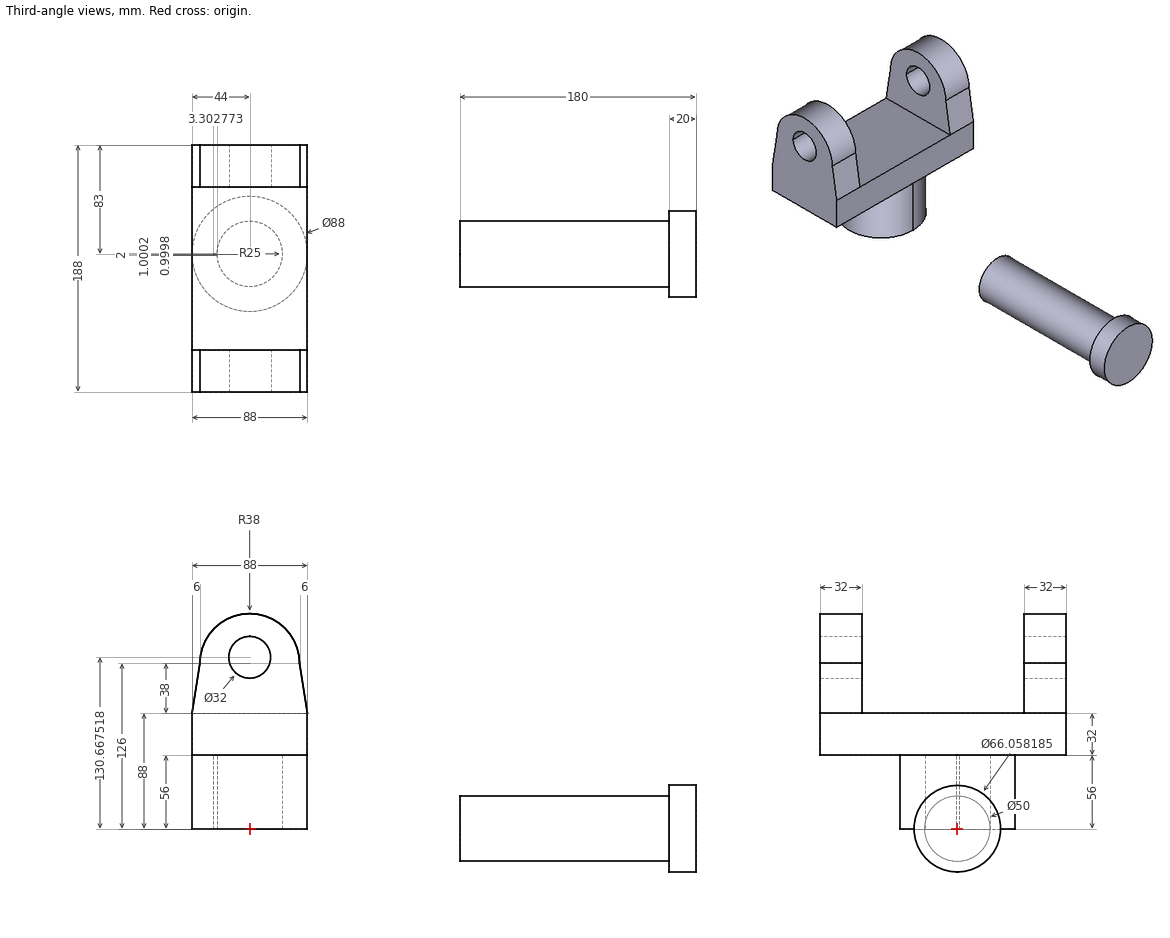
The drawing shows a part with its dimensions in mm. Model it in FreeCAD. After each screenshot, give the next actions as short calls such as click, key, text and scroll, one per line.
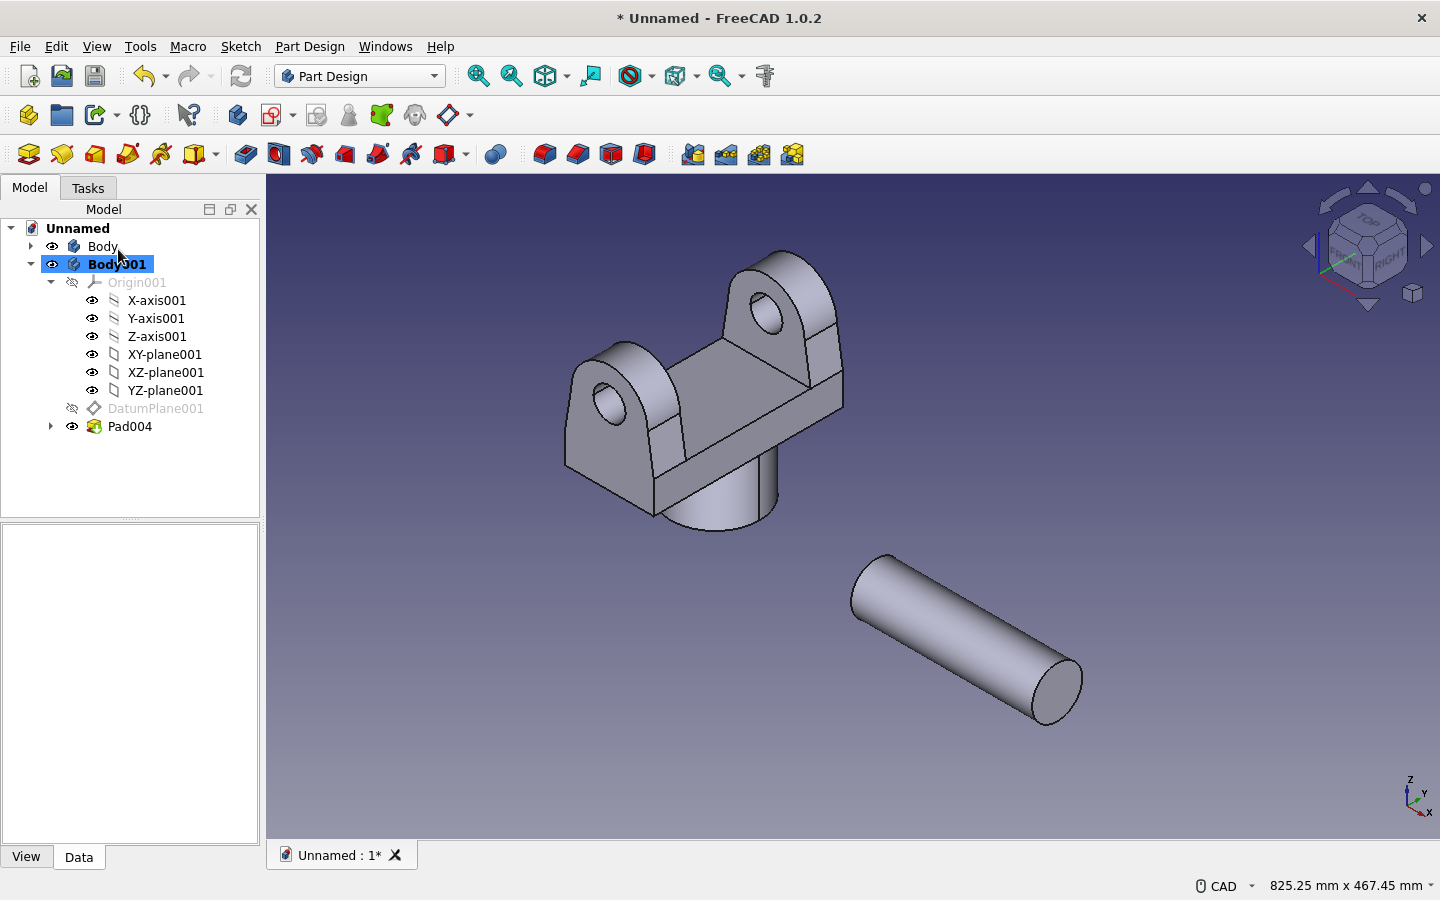
click(1057, 691)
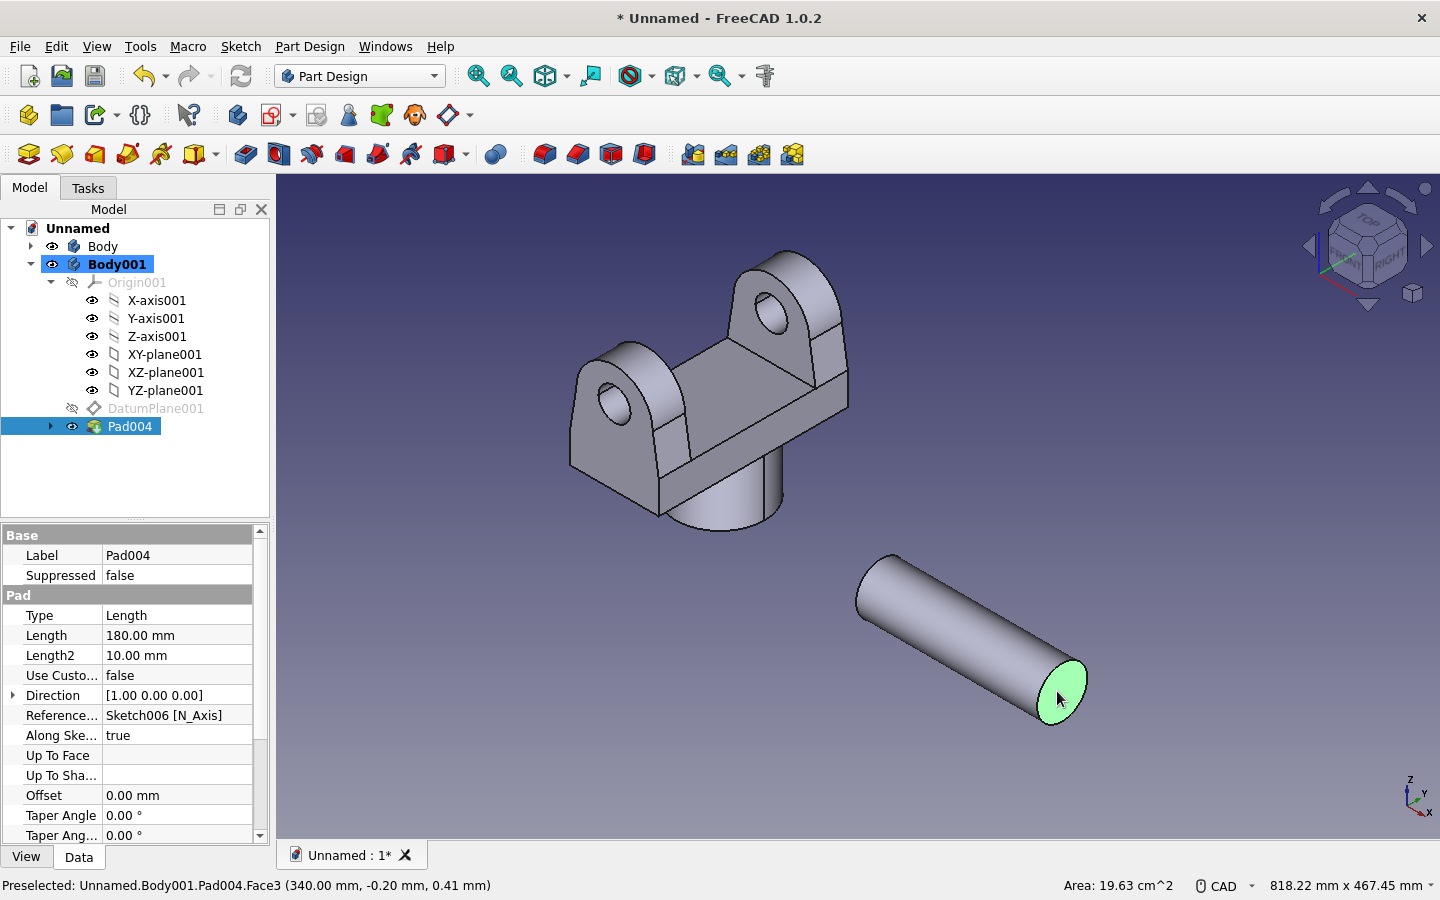
click(270, 116)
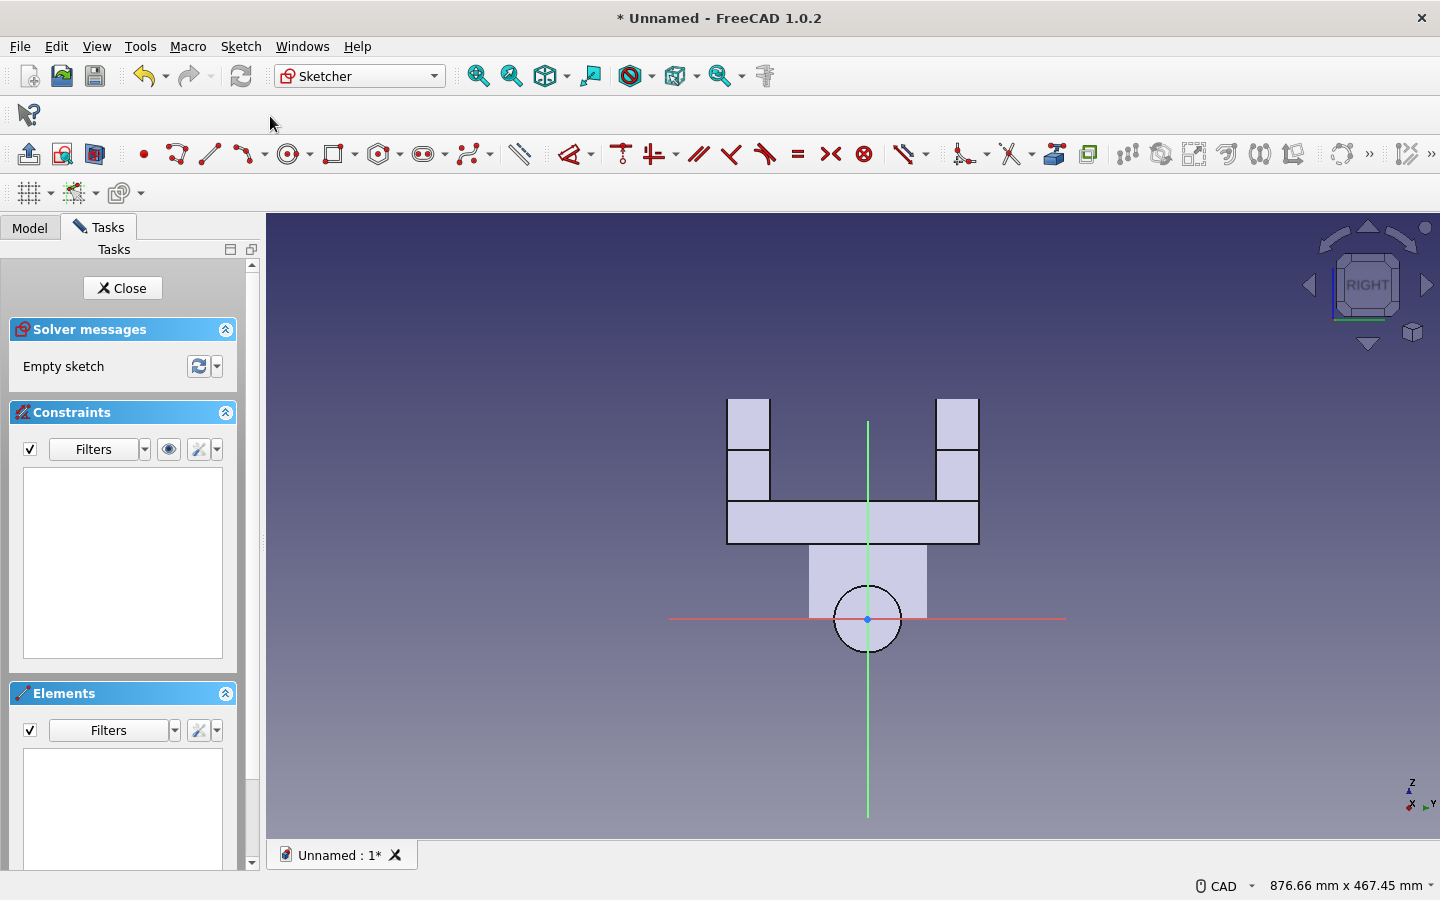
scroll(889, 643, up, 8)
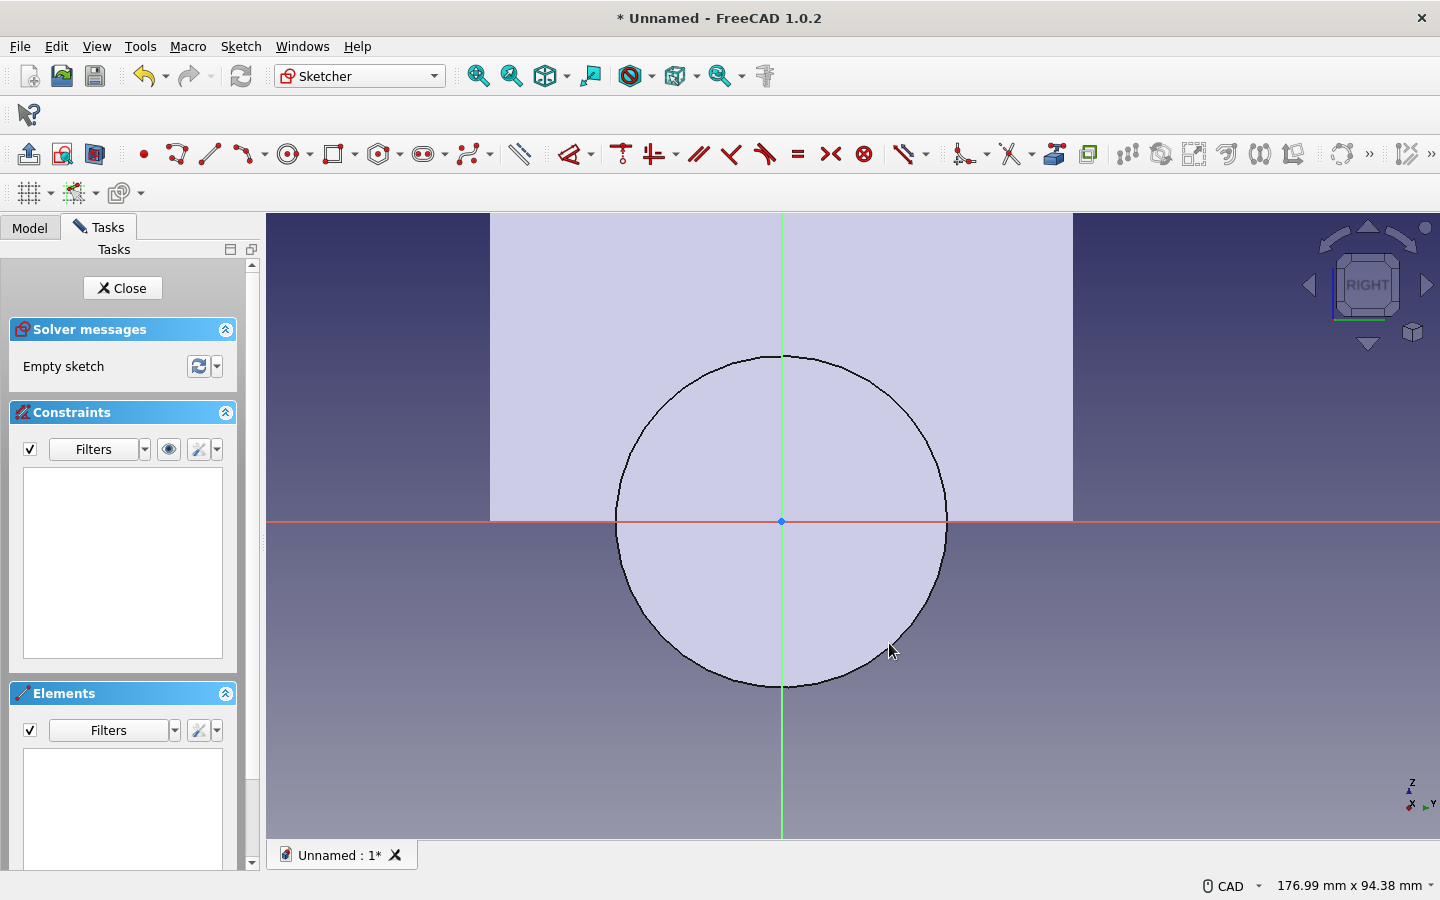
key(g)
key(c)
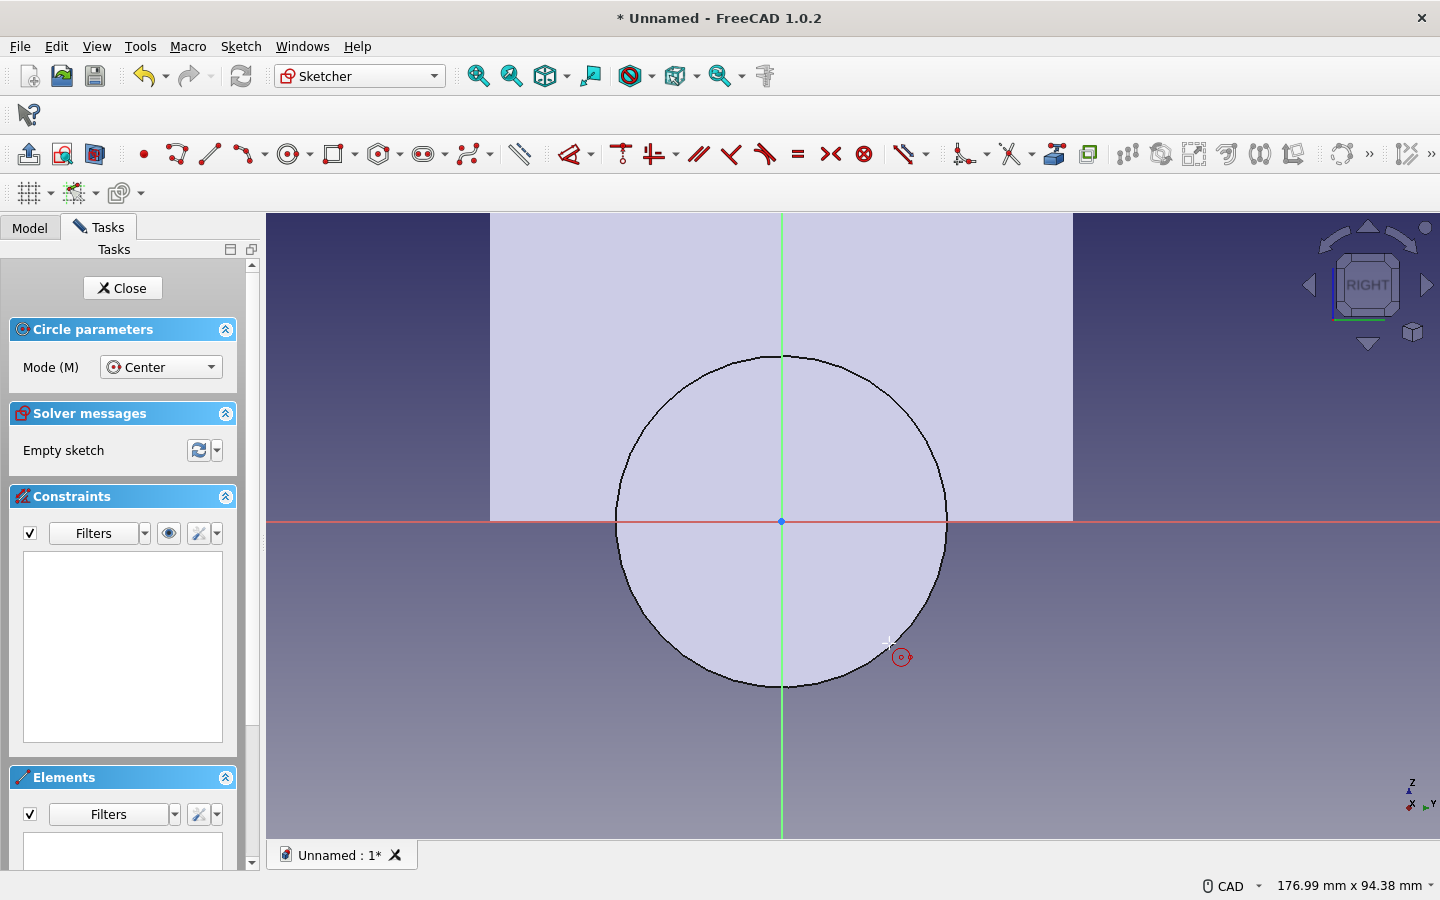
click(782, 522)
click(936, 367)
key(Escape)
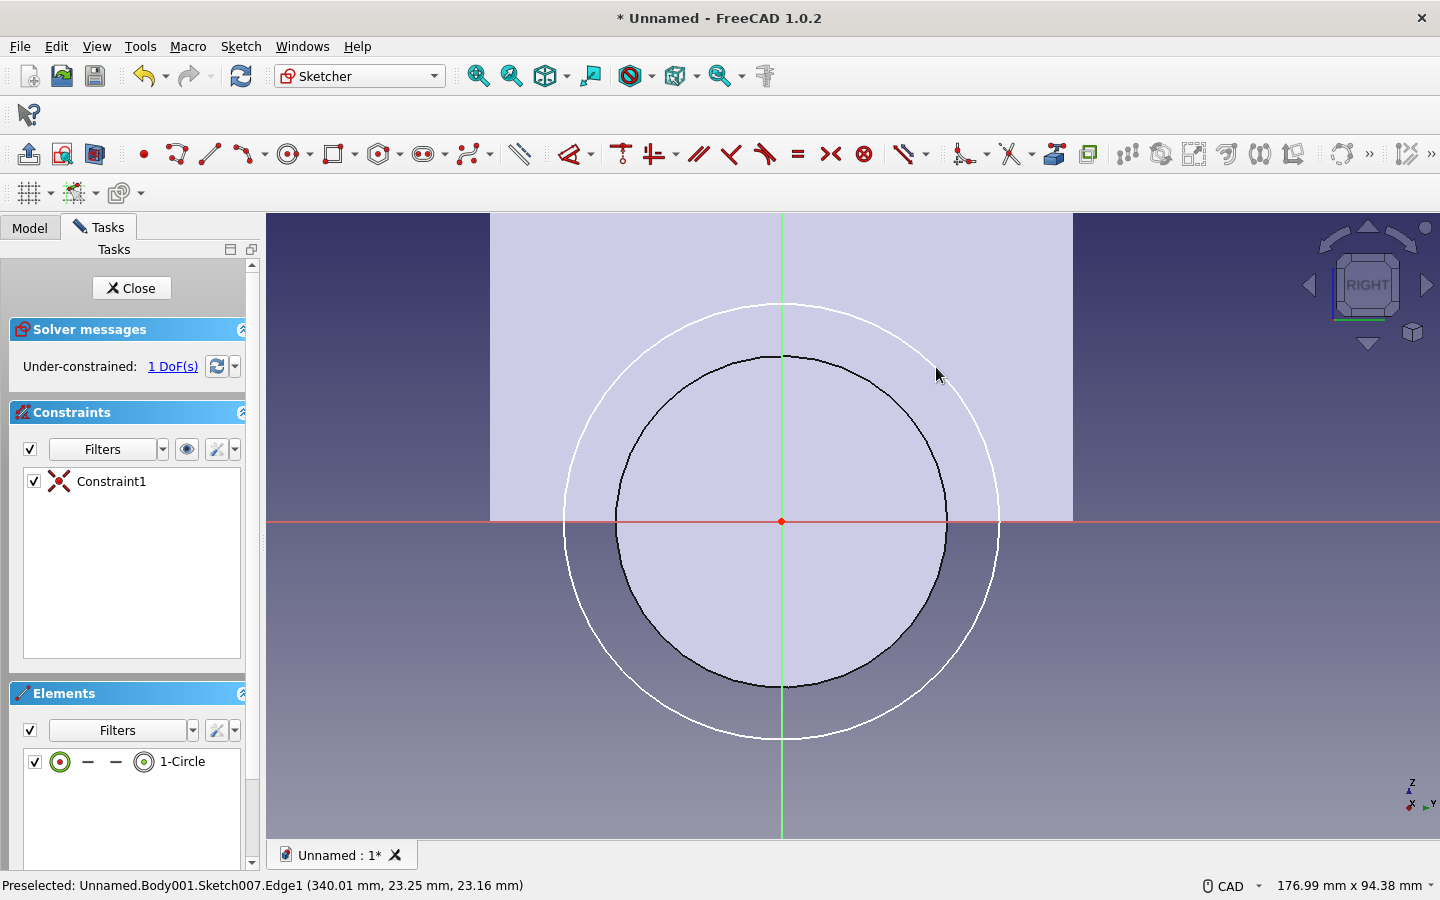
key(d)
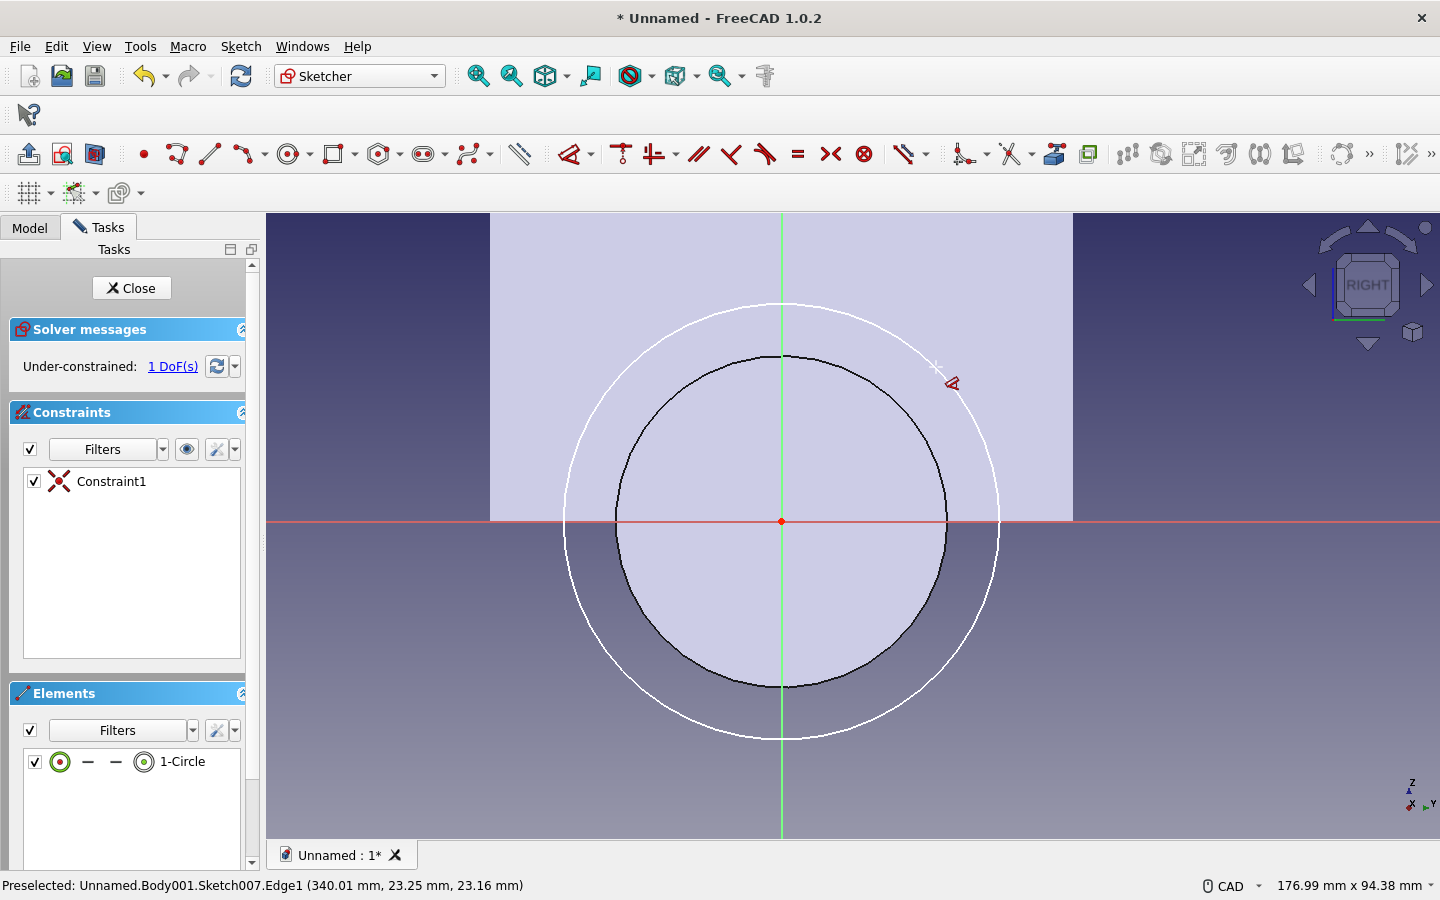
click(935, 367)
click(958, 344)